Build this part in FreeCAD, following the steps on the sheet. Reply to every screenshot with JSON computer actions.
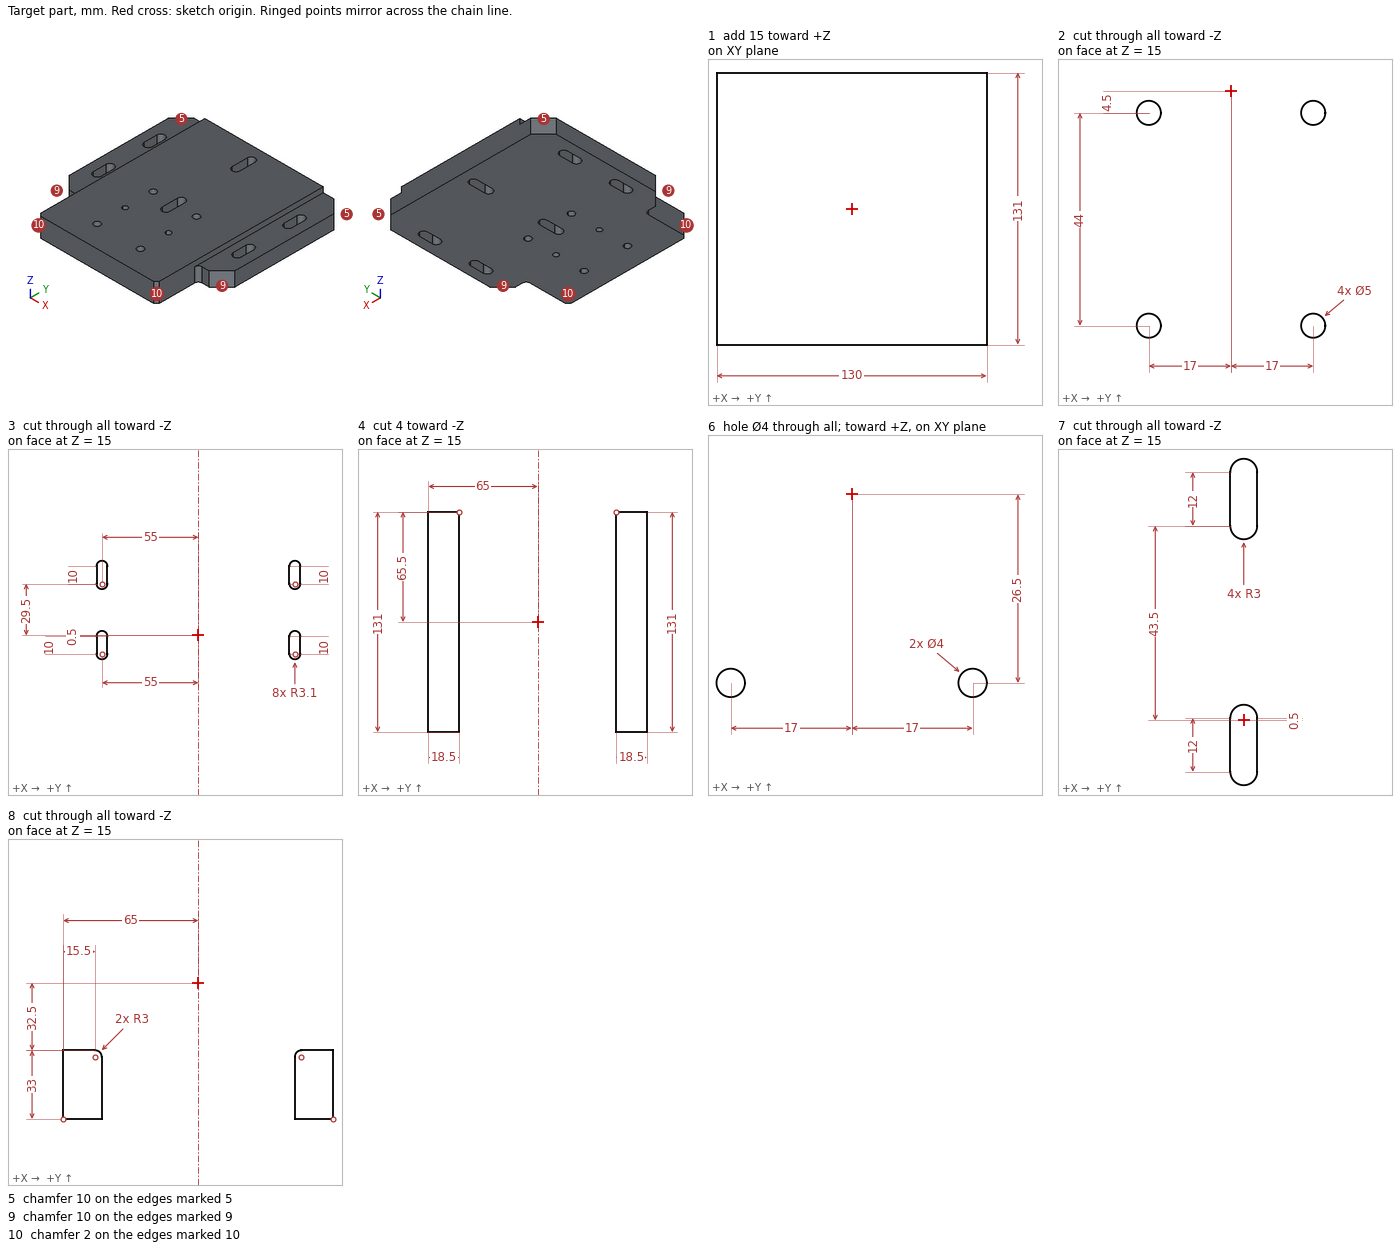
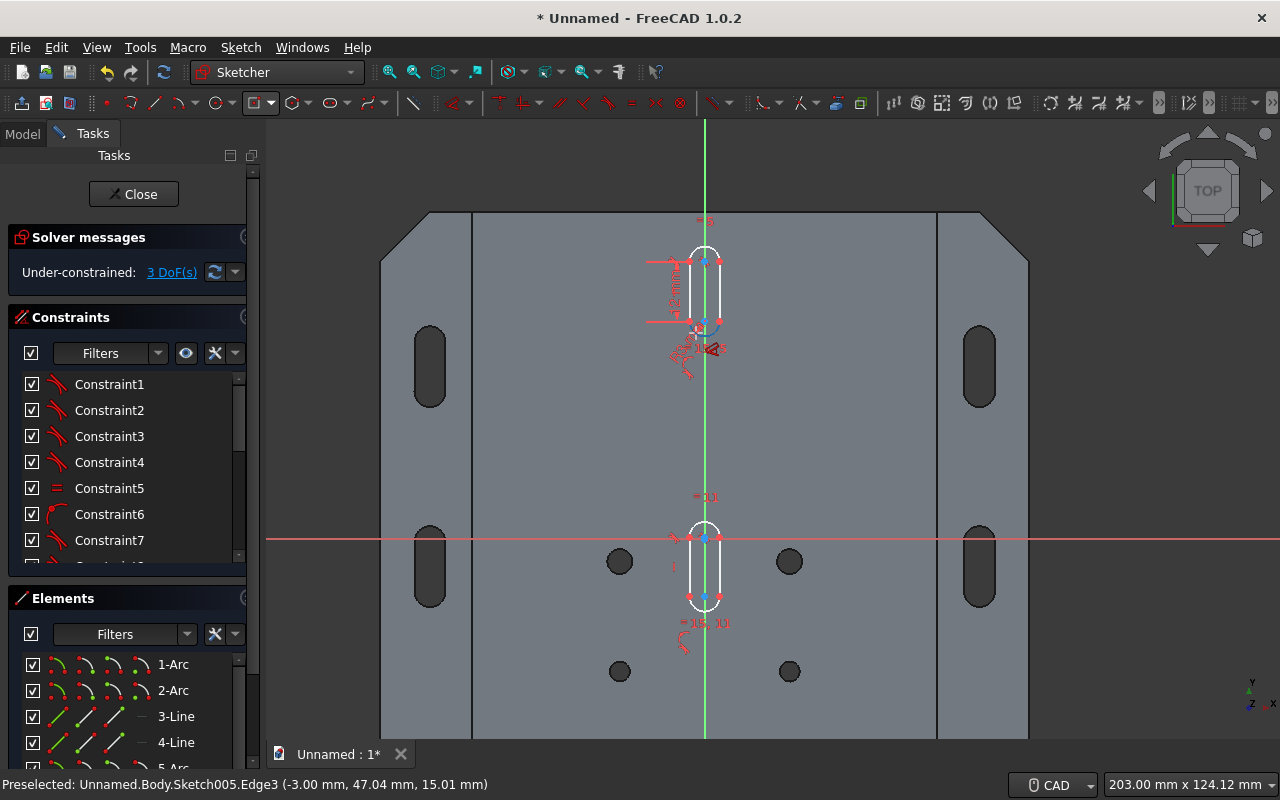
{"action": "left_click", "coordinate": [690, 579]}
{"action": "left_click", "coordinate": [656, 567]}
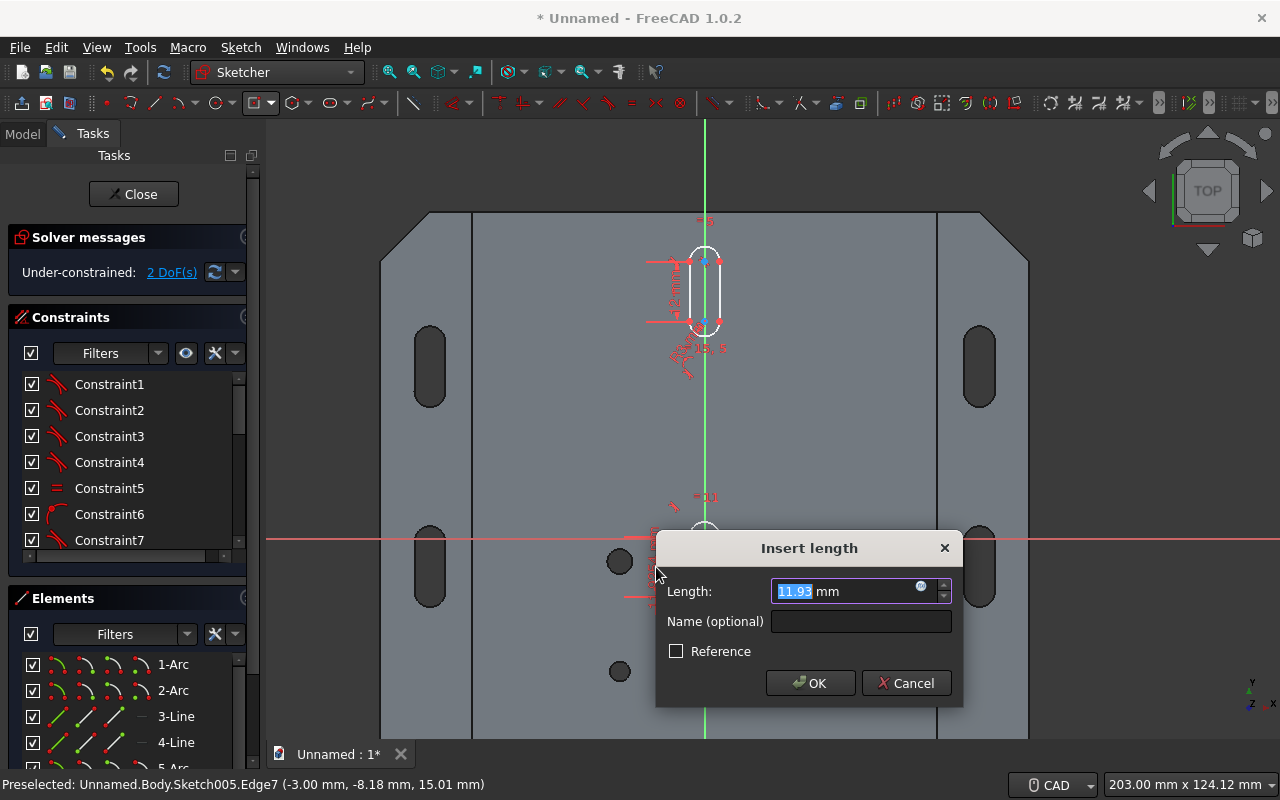
{"action": "type", "text": "12"}
{"action": "key", "text": "Return"}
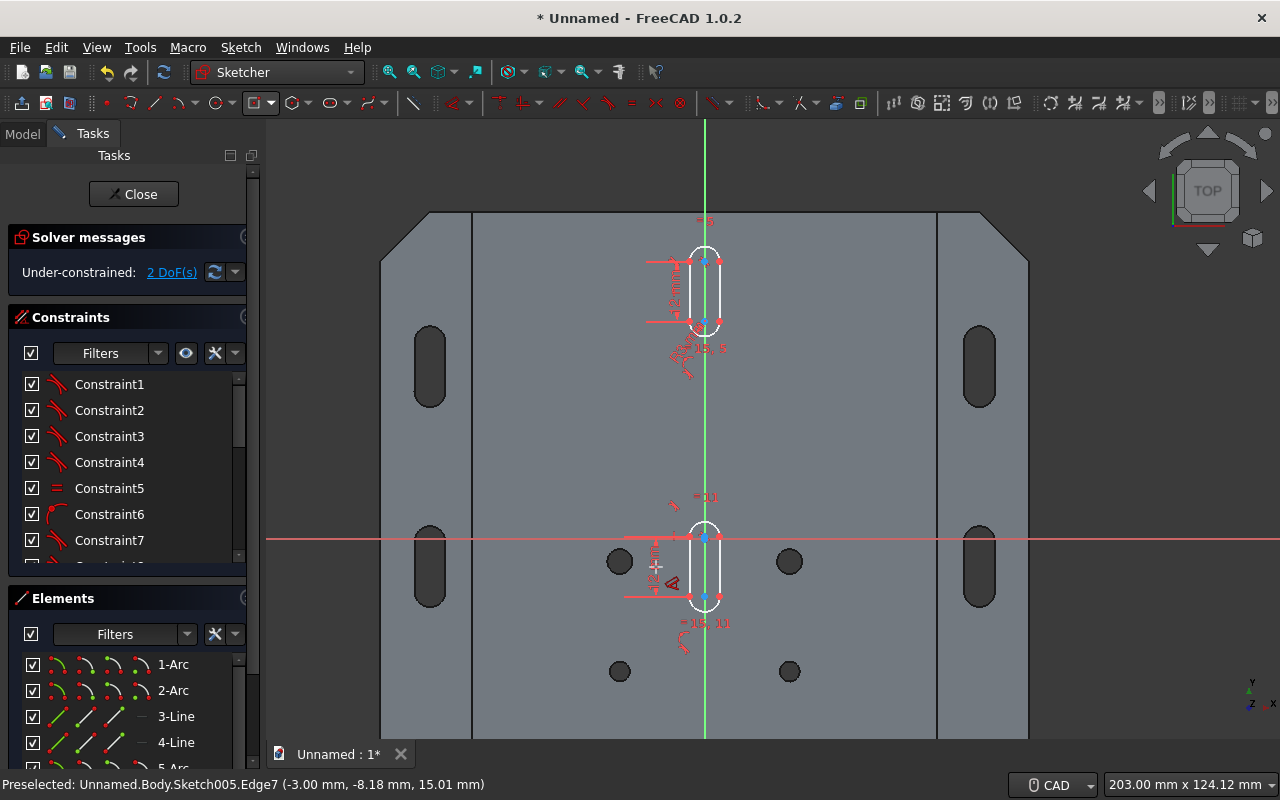
{"action": "scroll", "coordinate": [720, 537], "scroll_direction": "up", "scroll_amount": 14}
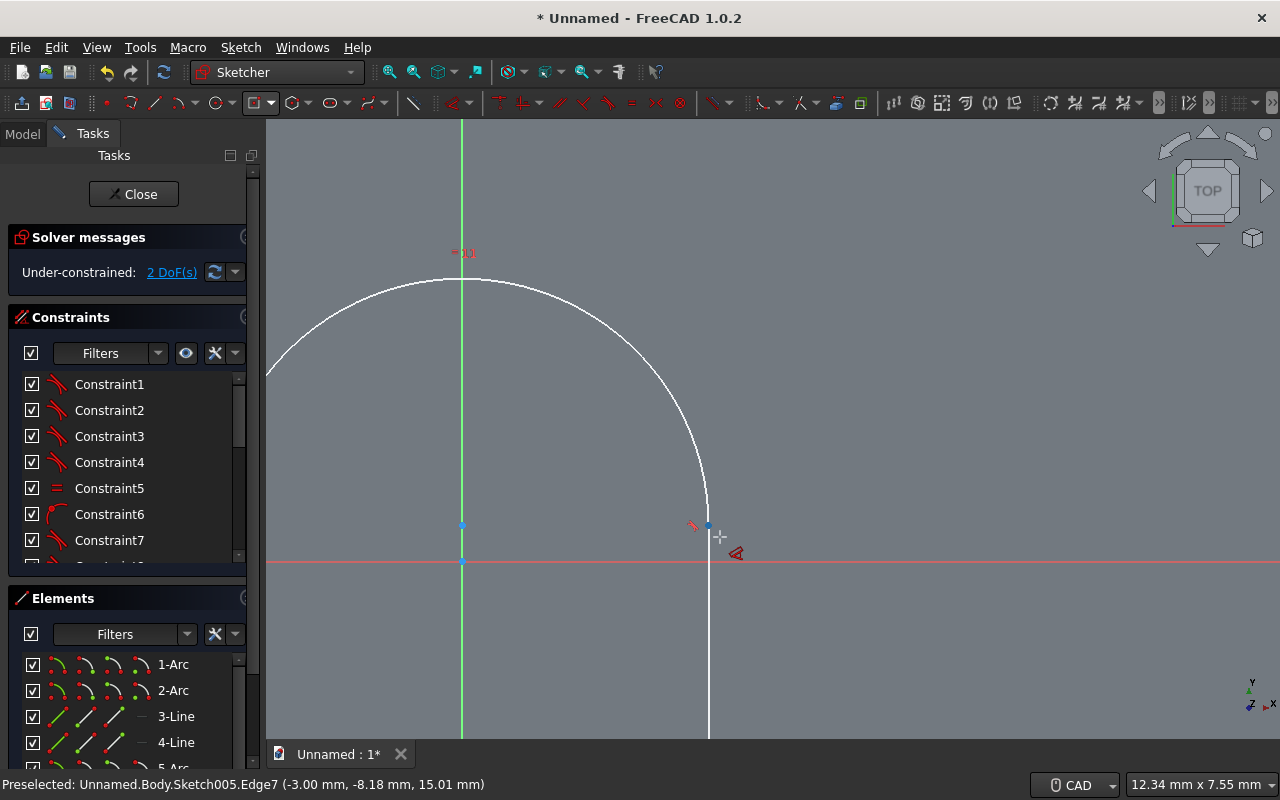
{"action": "left_click", "coordinate": [709, 525]}
{"action": "left_click", "coordinate": [743, 543]}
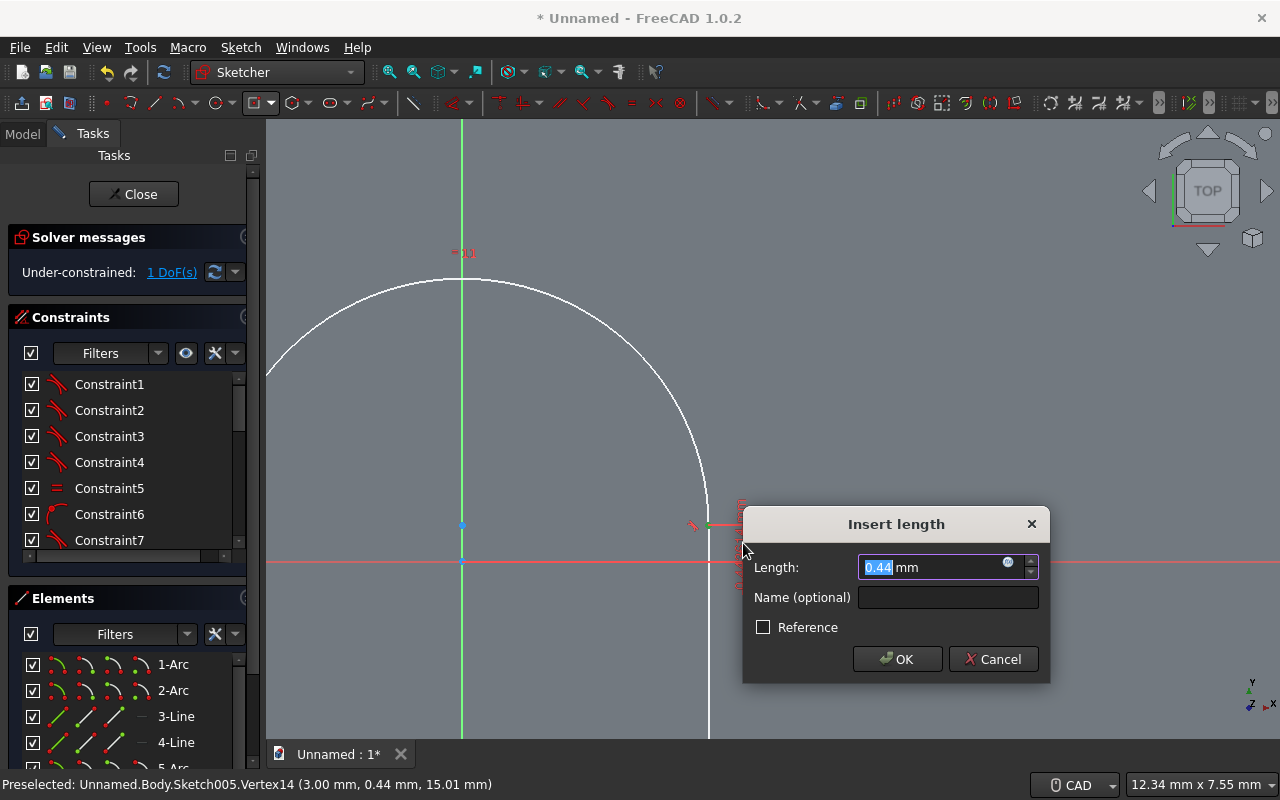
{"action": "type", "text": "0.5"}
{"action": "key", "text": "Return"}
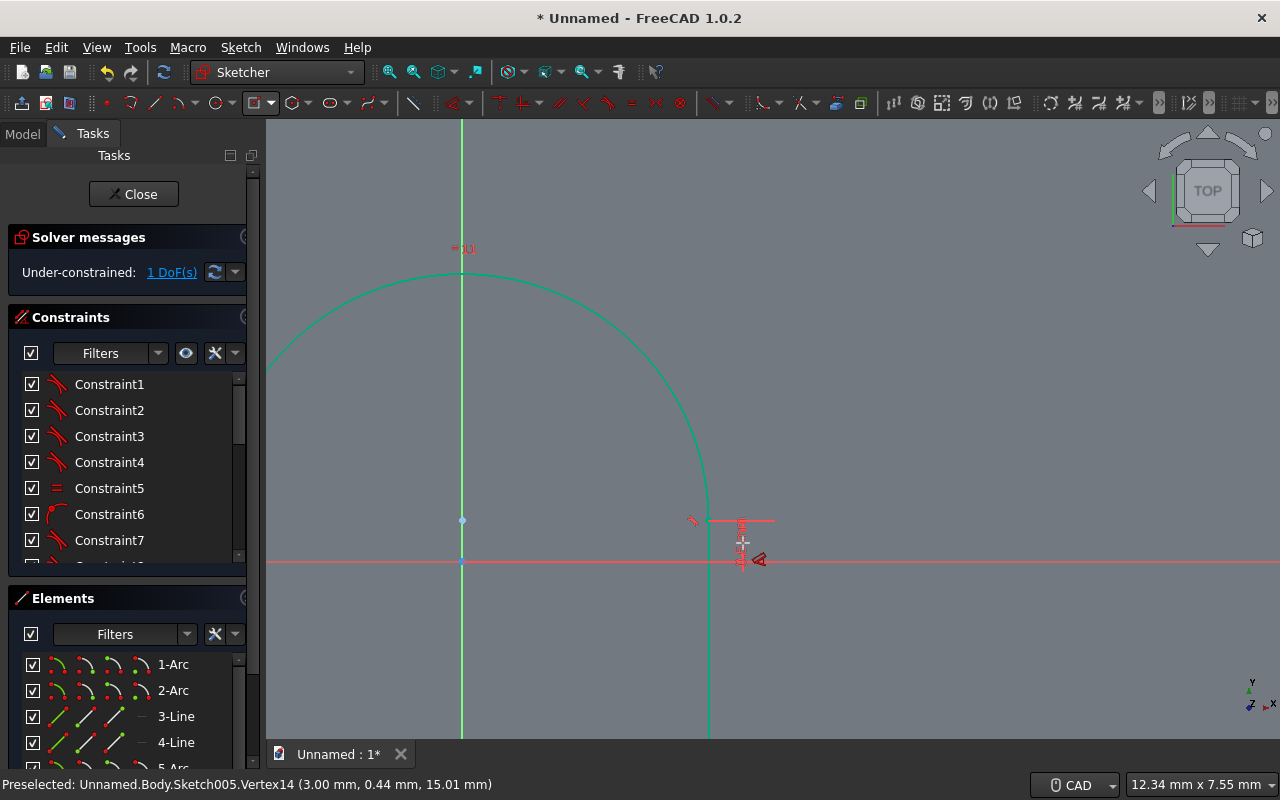
{"action": "scroll", "coordinate": [720, 537], "scroll_direction": "down", "scroll_amount": 14}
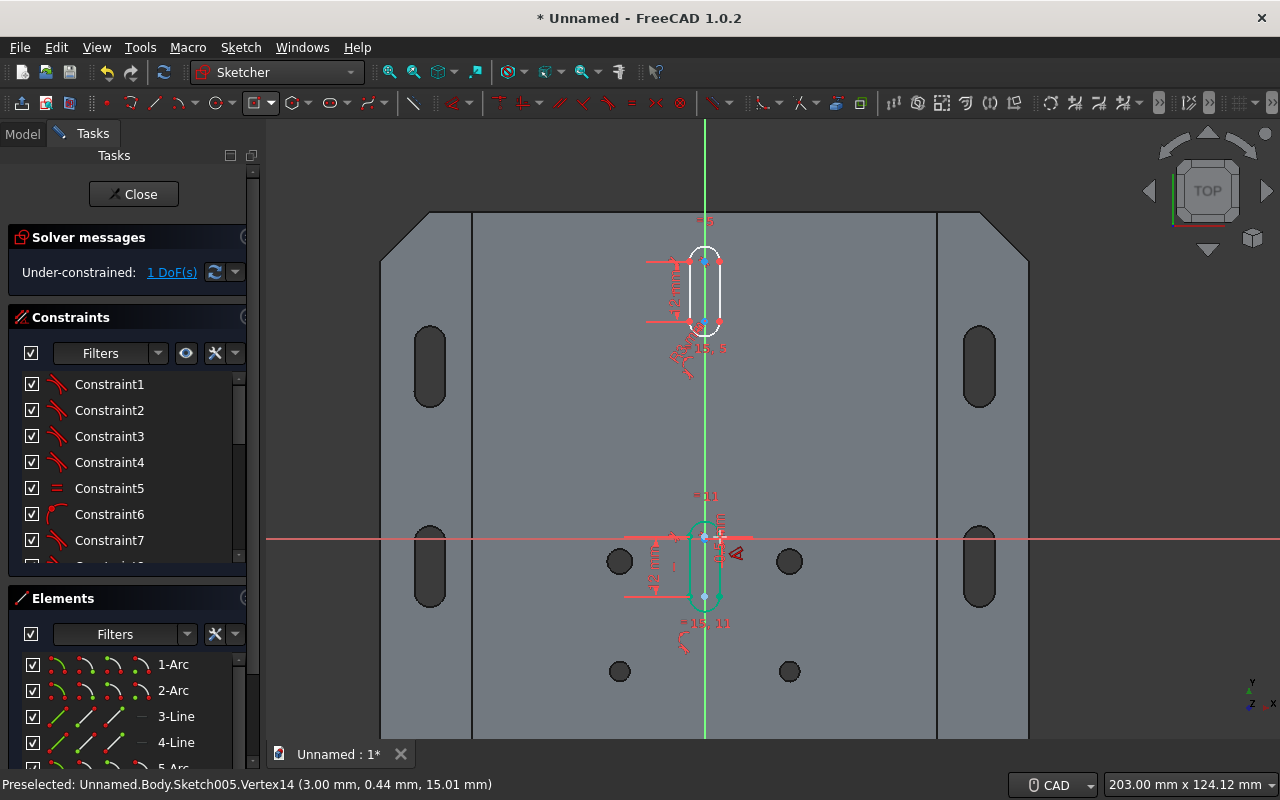
{"action": "left_click", "coordinate": [690, 322]}
{"action": "left_click", "coordinate": [656, 430]}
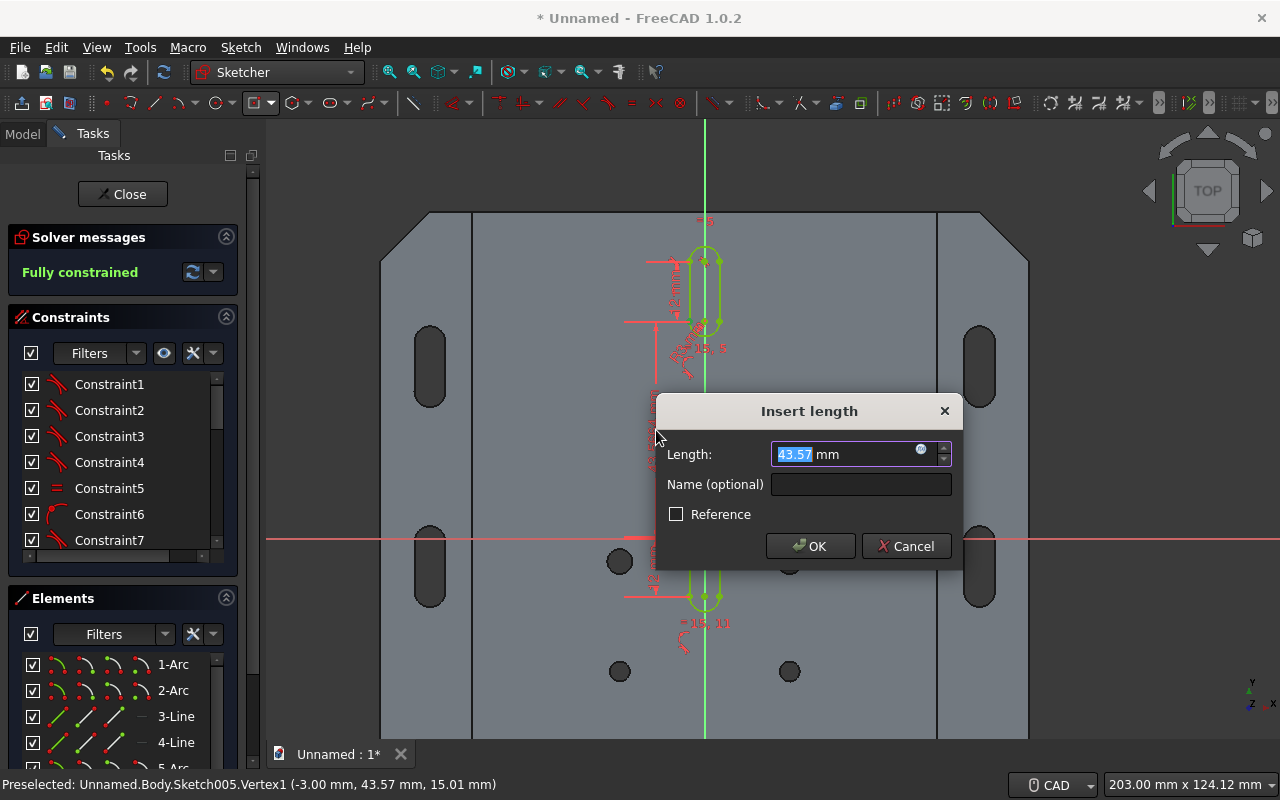
{"action": "type", "text": "43.5"}
{"action": "key", "text": "Return"}
{"action": "key", "text": "Escape"}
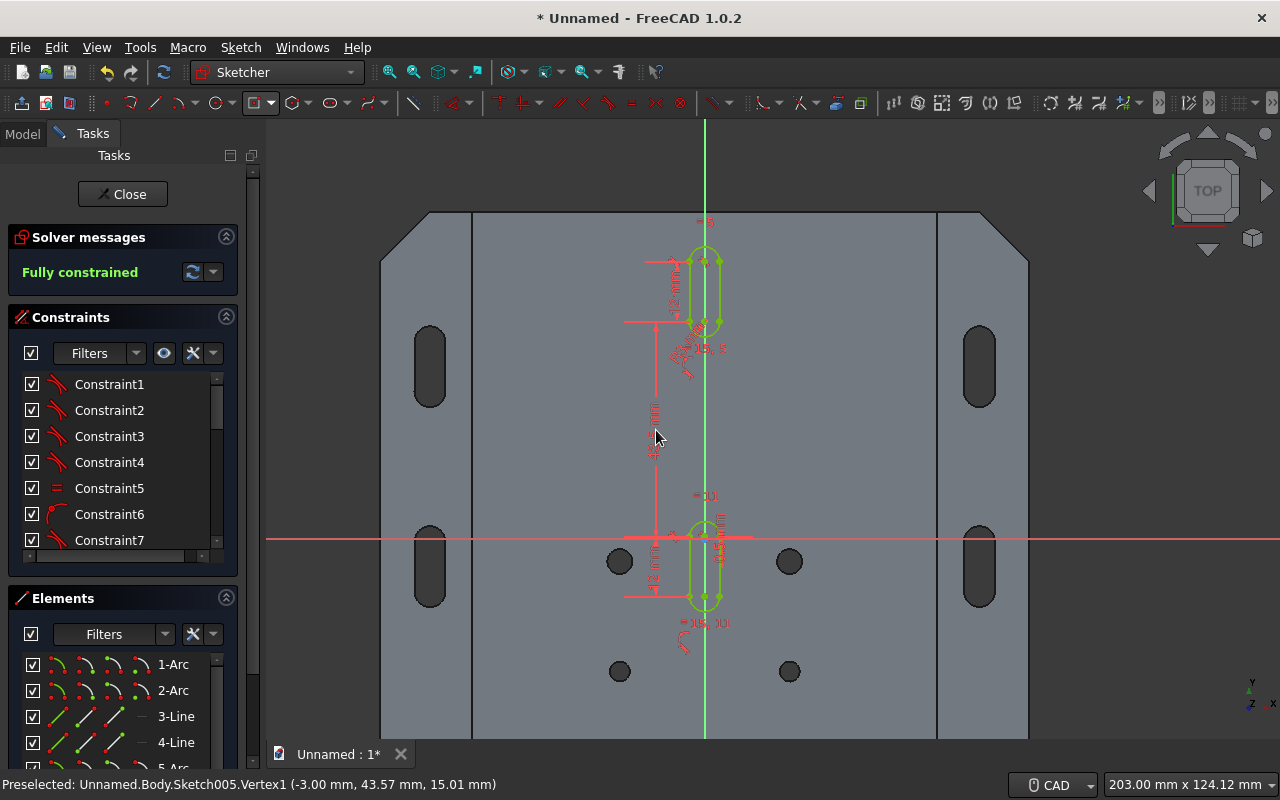
{"action": "left_click", "coordinate": [123, 194]}